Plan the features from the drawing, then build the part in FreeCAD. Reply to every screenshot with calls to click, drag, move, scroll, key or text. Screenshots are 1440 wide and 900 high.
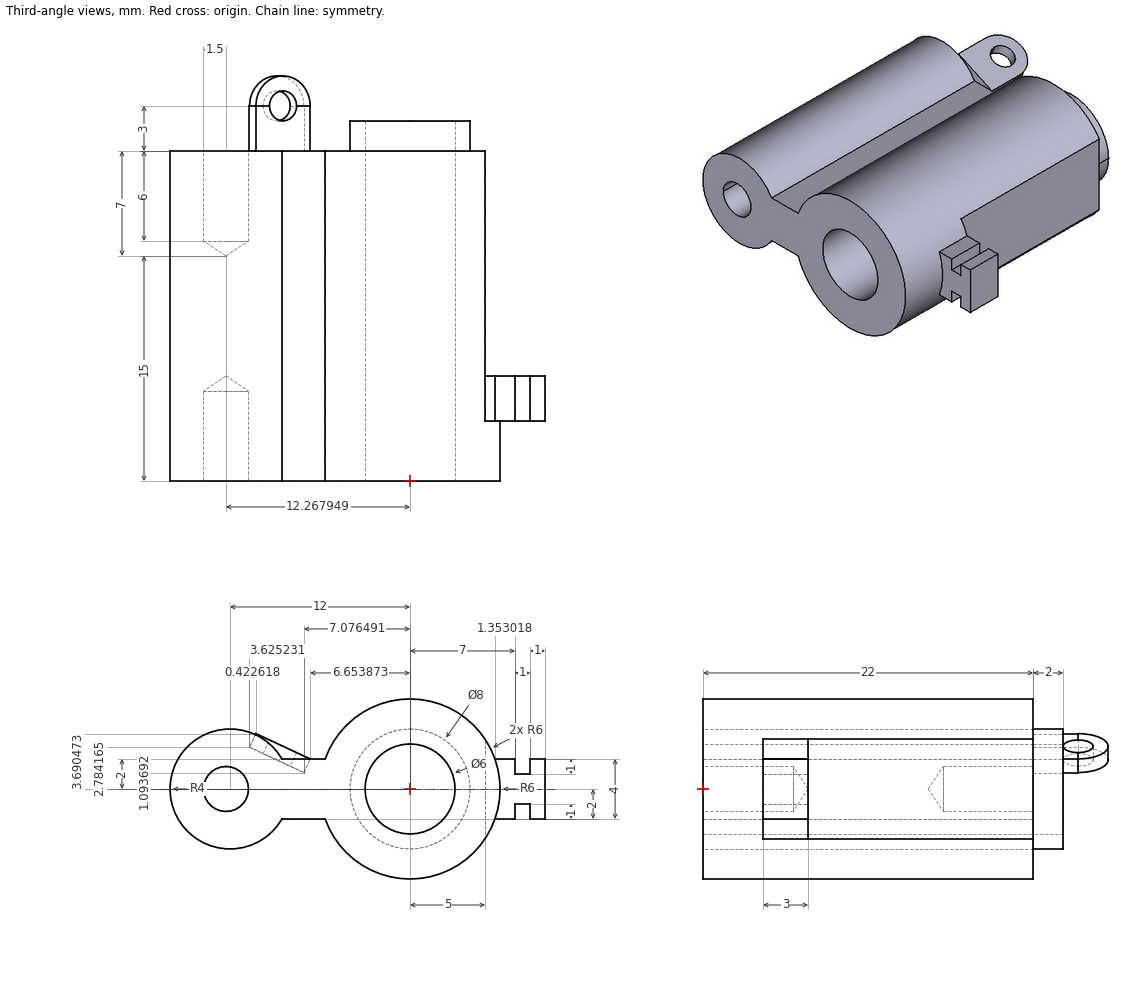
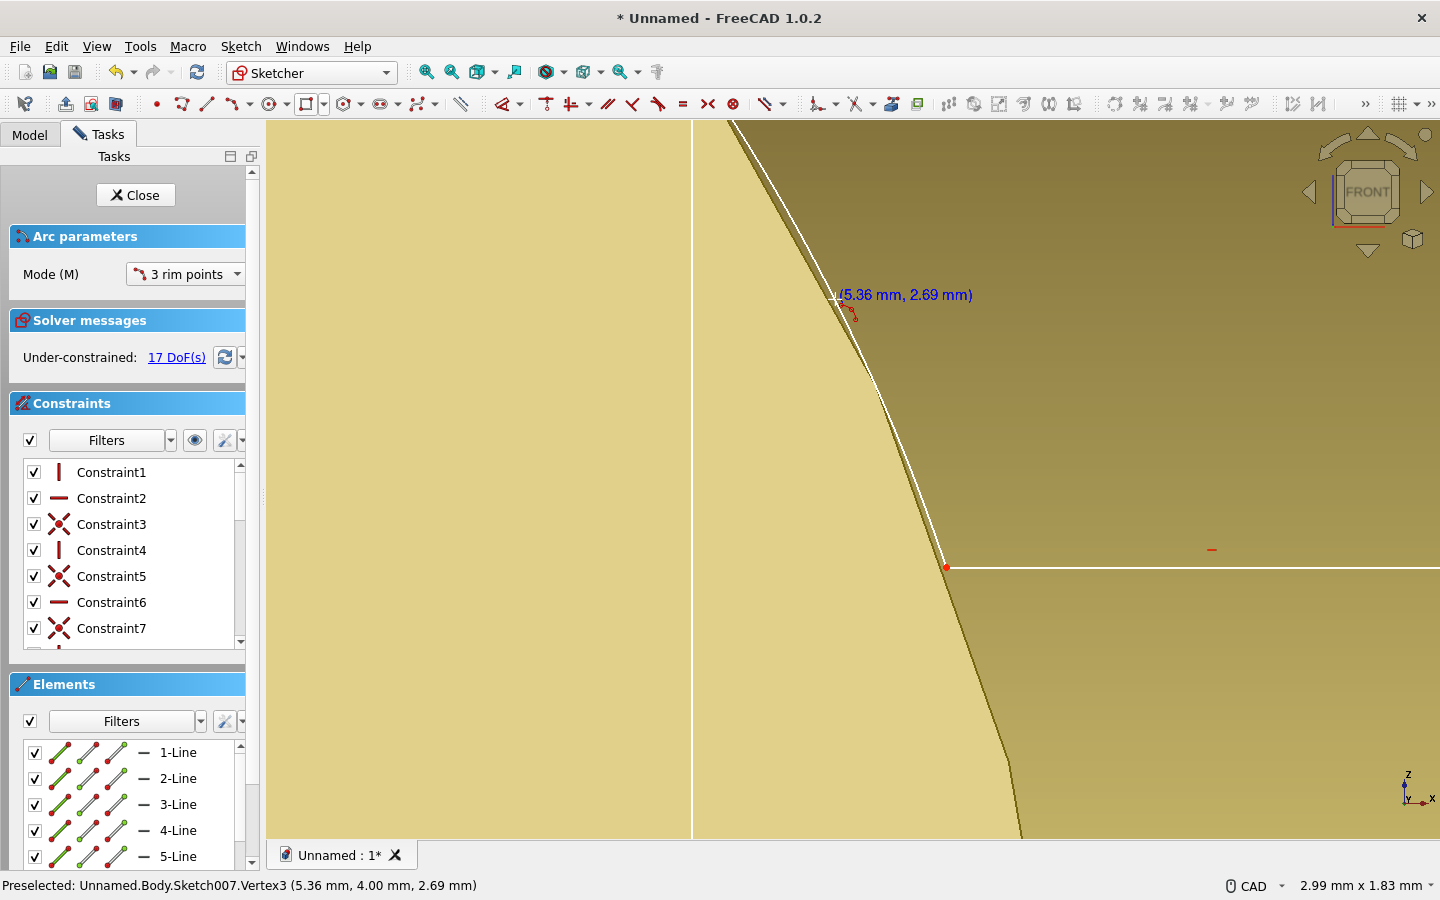
scroll(842, 306, down, 9)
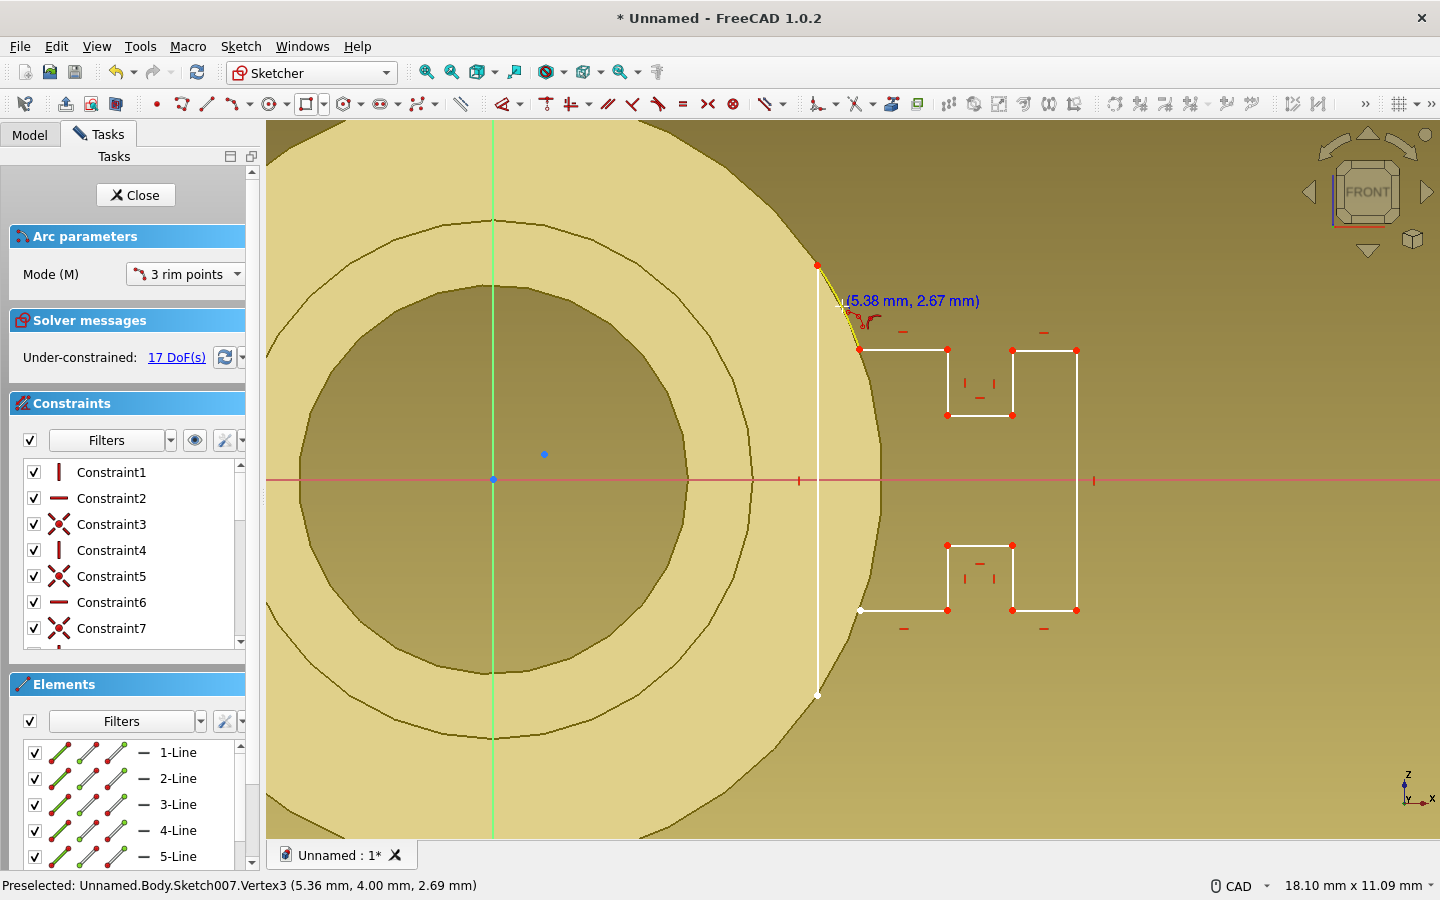
click(861, 611)
click(818, 696)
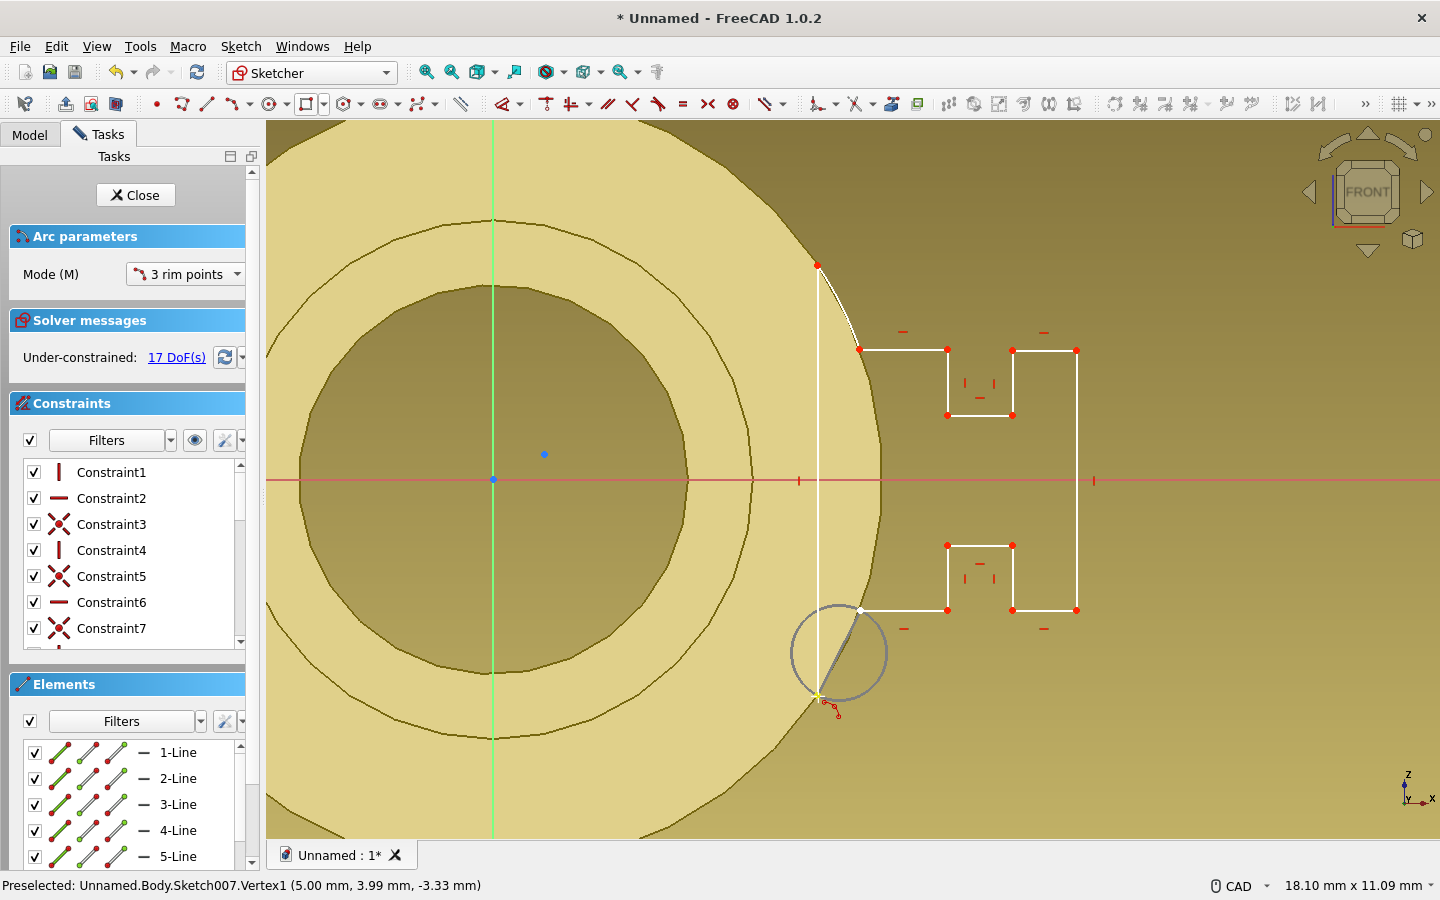
scroll(842, 653, up, 9)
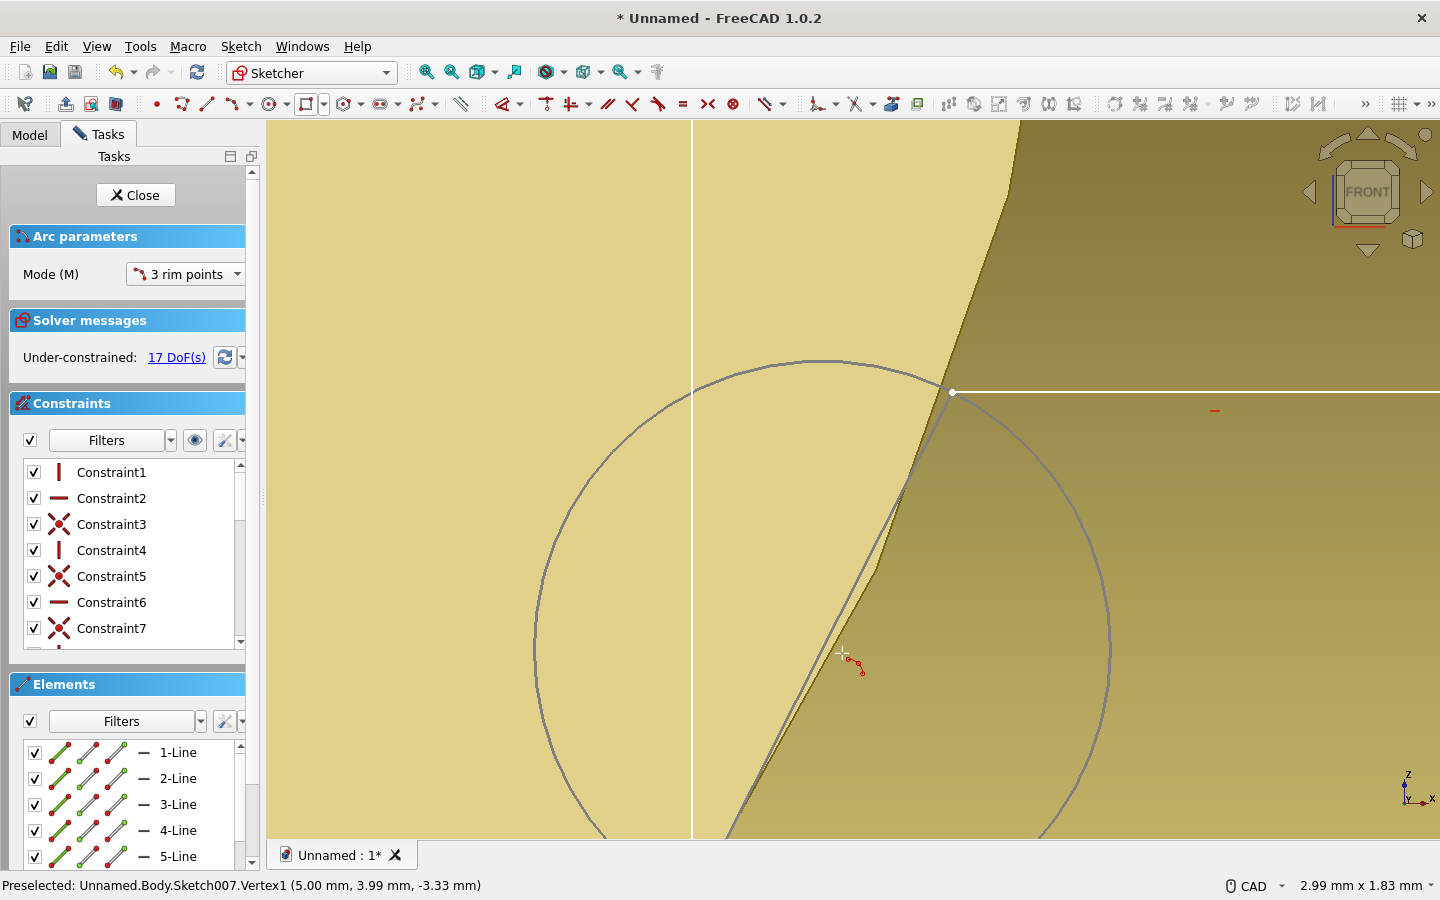
click(837, 652)
key(Escape)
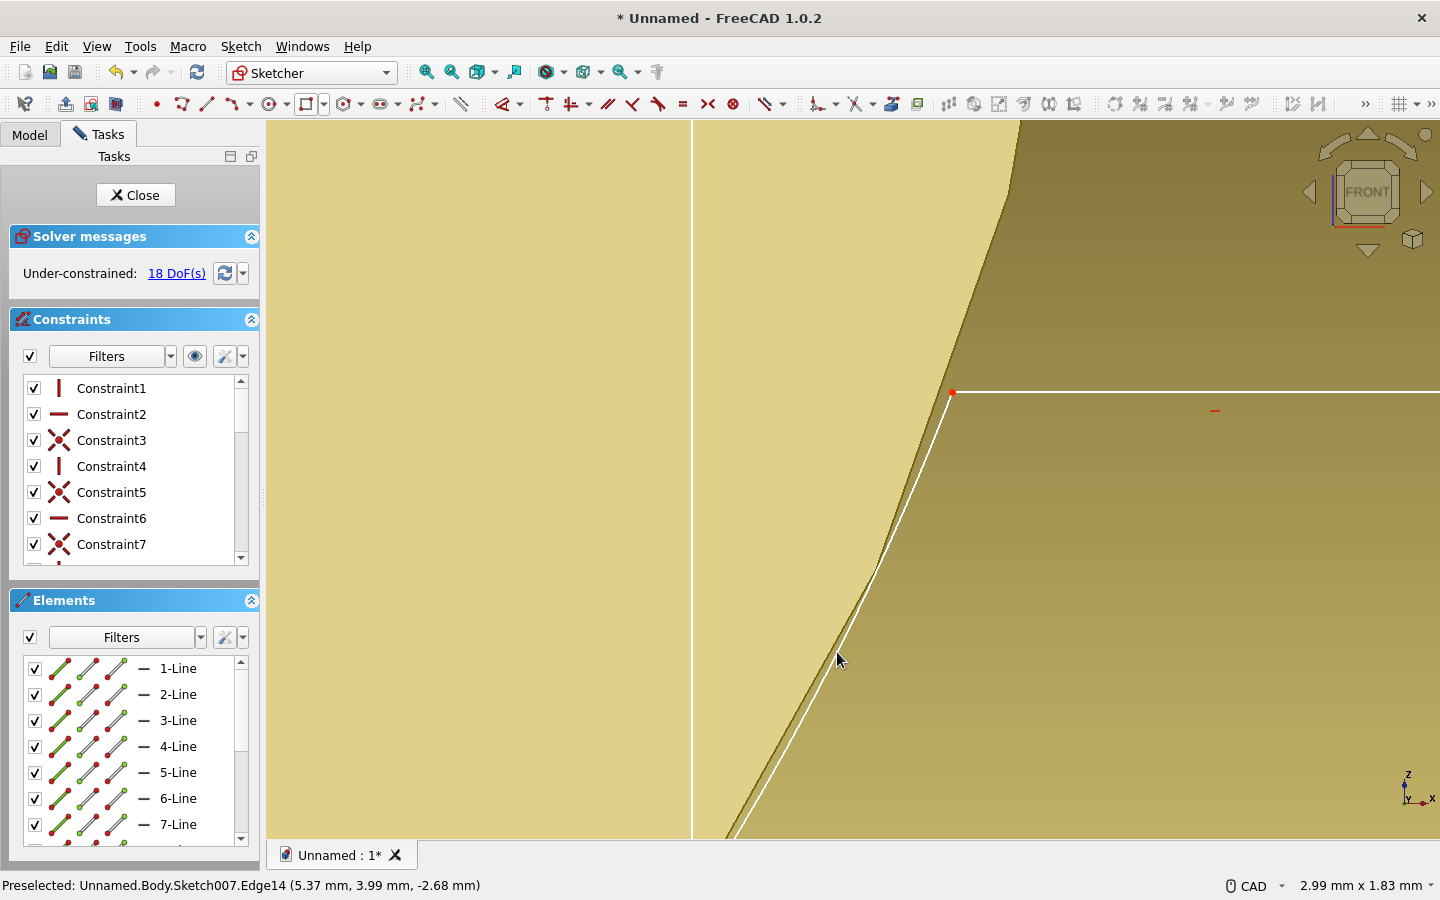
scroll(842, 654, down, 9)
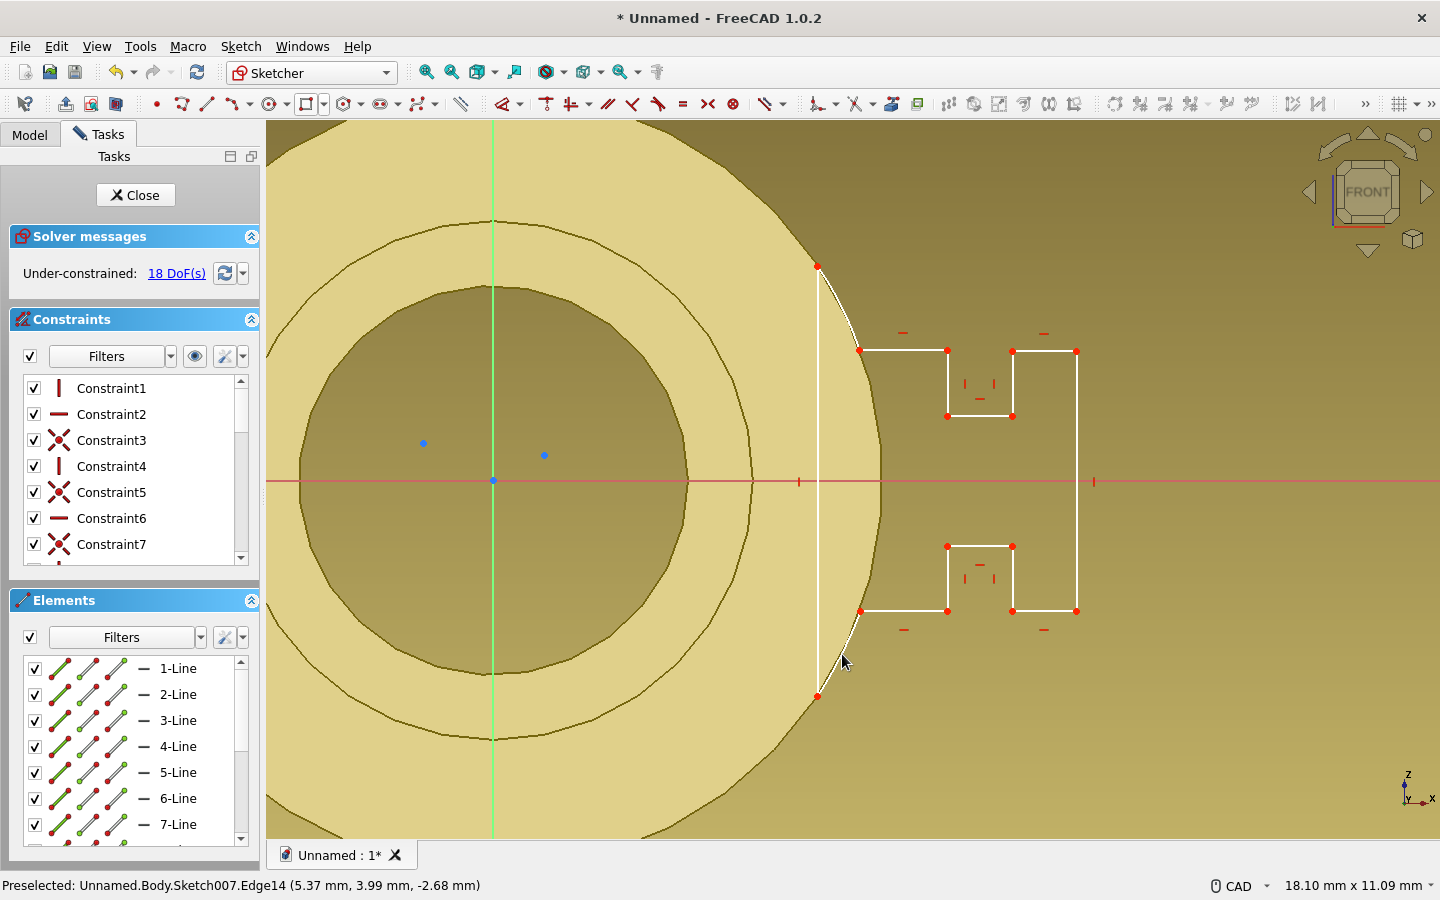
click(850, 324)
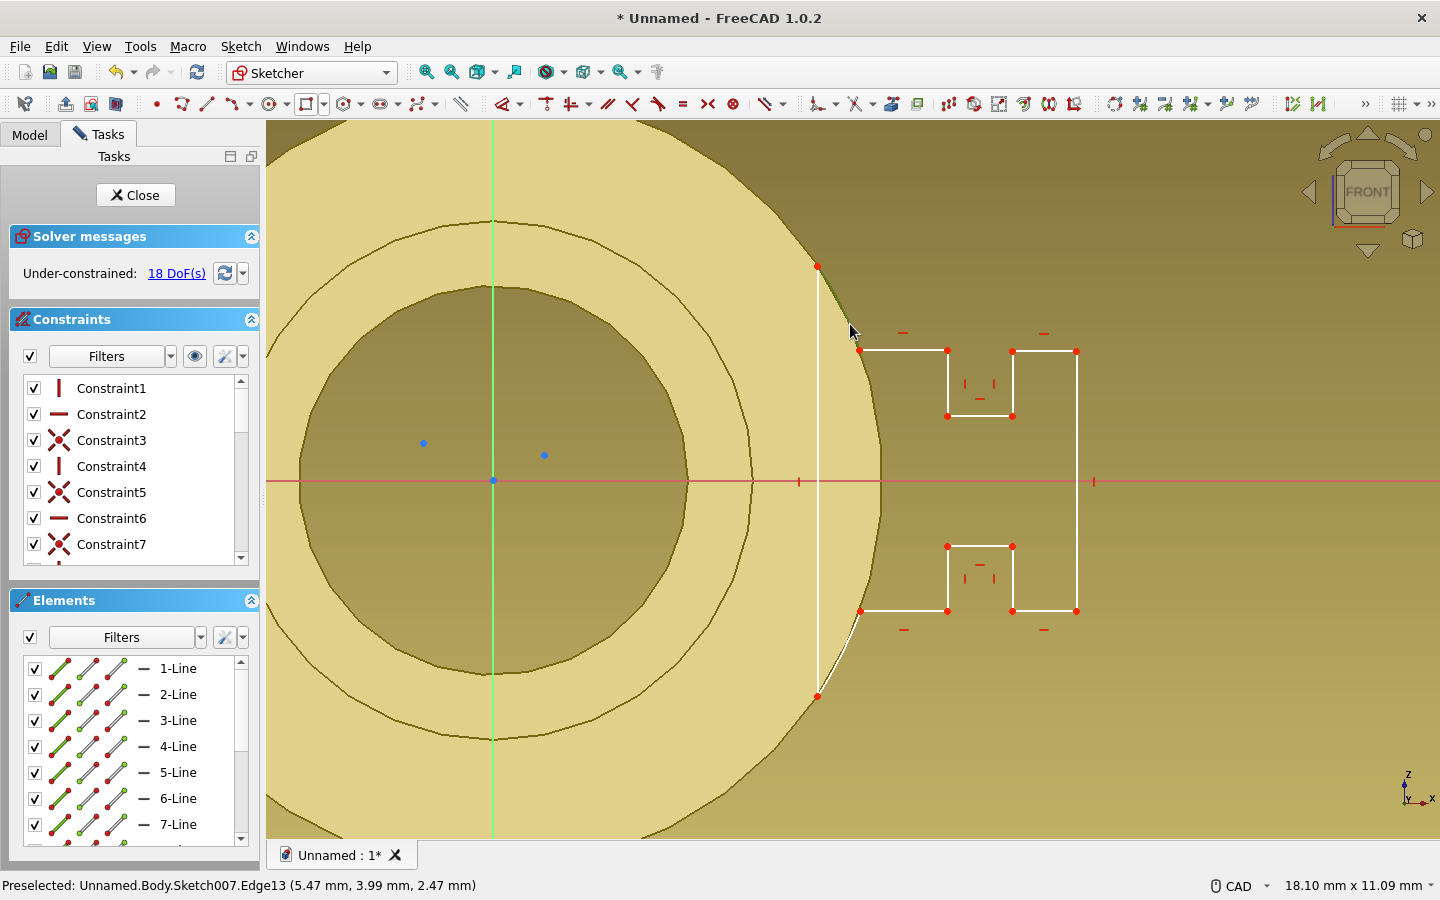
click(832, 672)